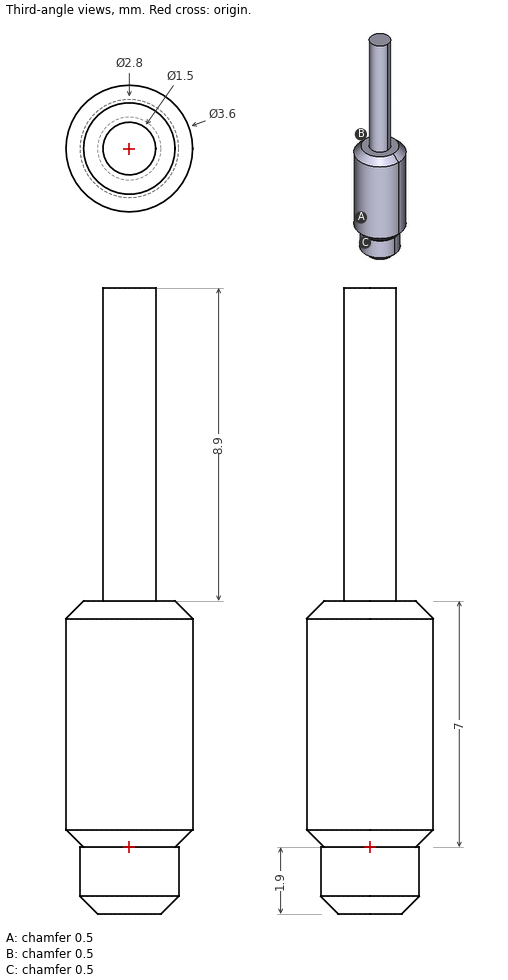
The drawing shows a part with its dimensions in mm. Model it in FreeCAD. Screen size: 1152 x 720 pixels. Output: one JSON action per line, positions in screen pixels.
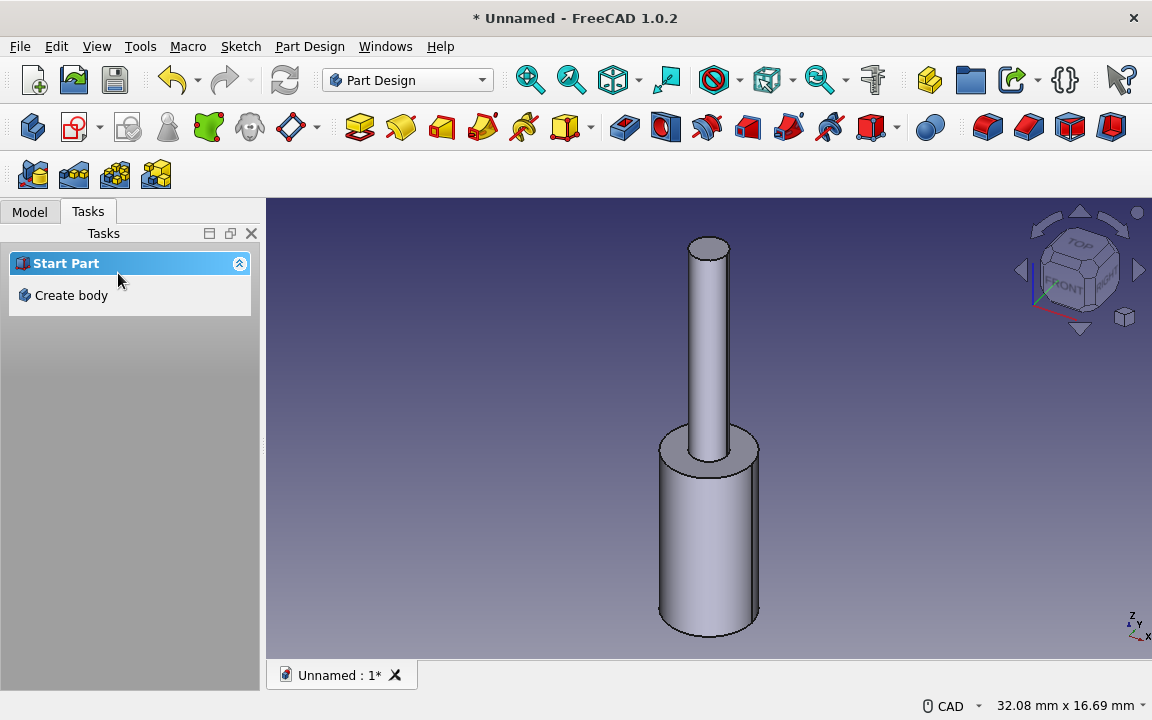
{"action": "key", "text": "0"}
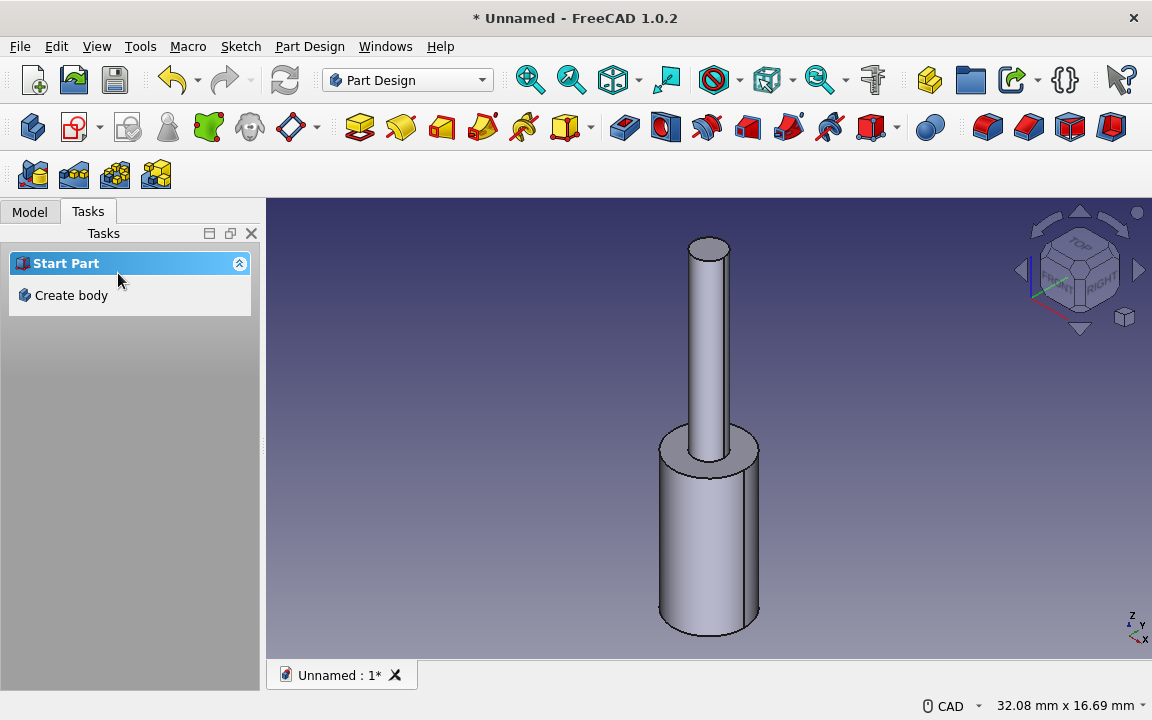
{"action": "key", "text": "2"}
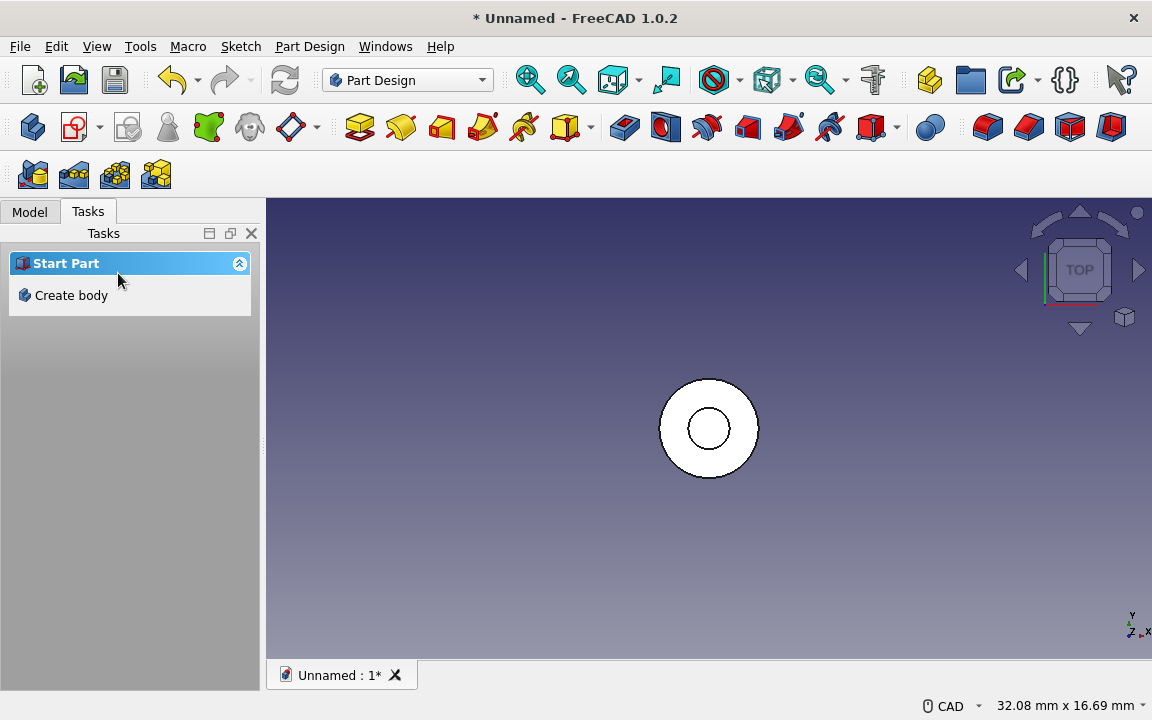
{"action": "key", "text": "v f"}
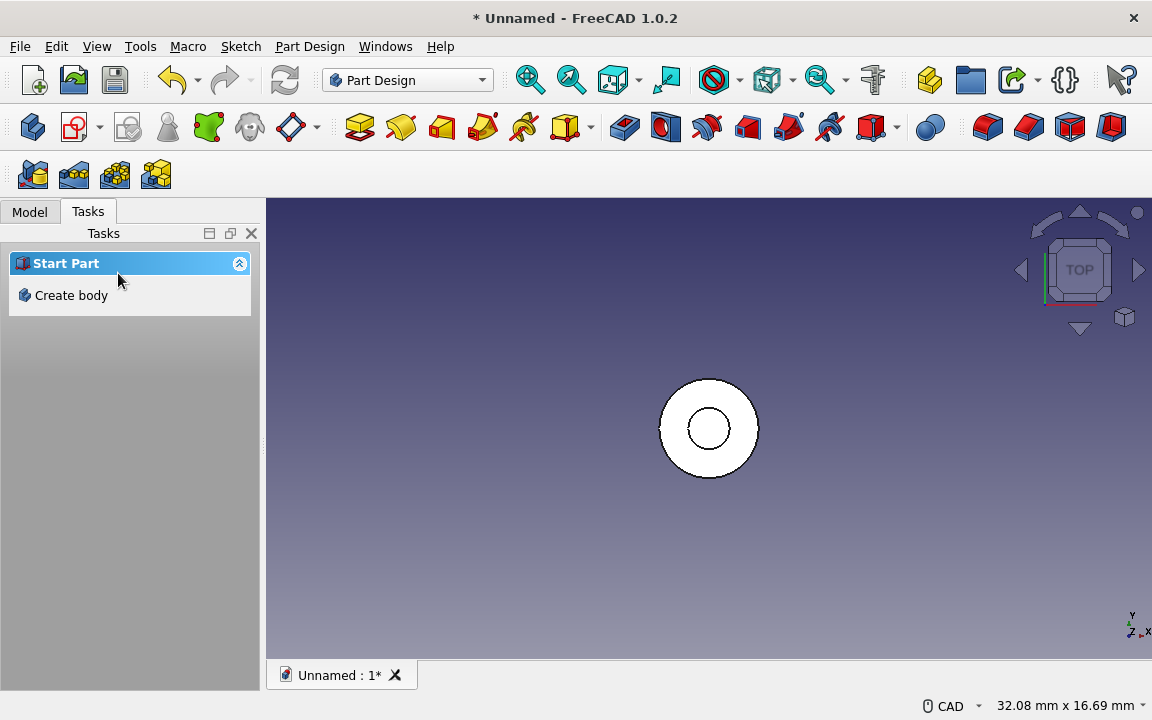
{"action": "key", "text": "1"}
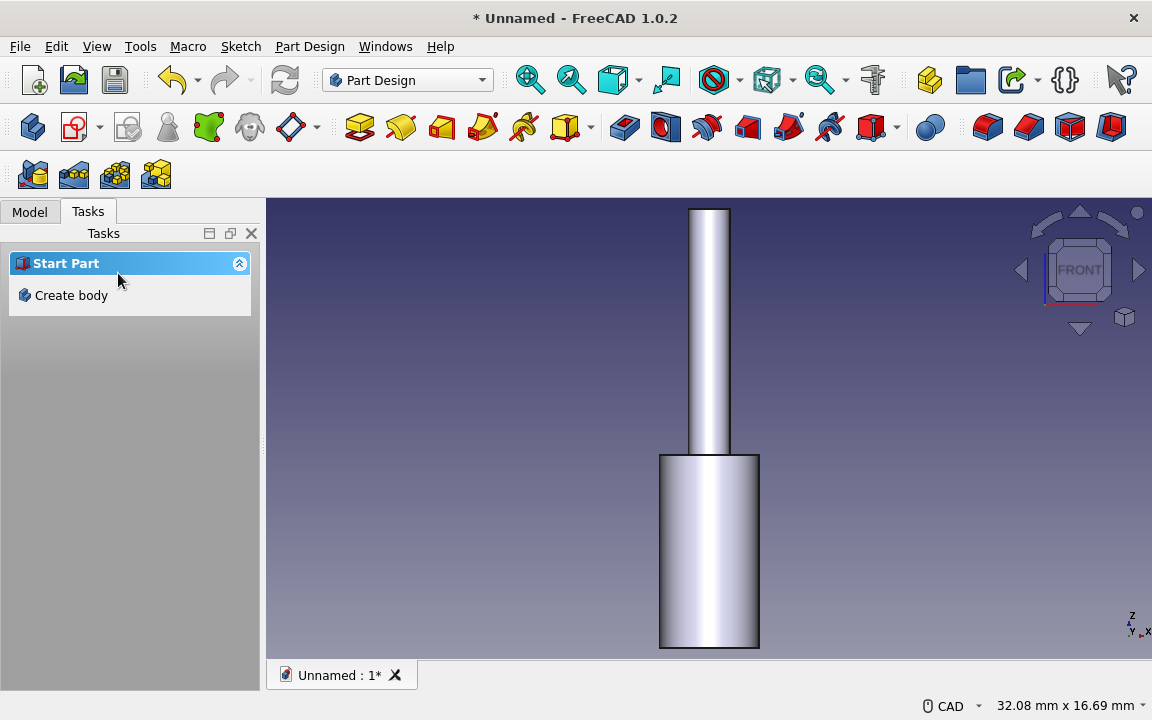
{"action": "key", "text": "3"}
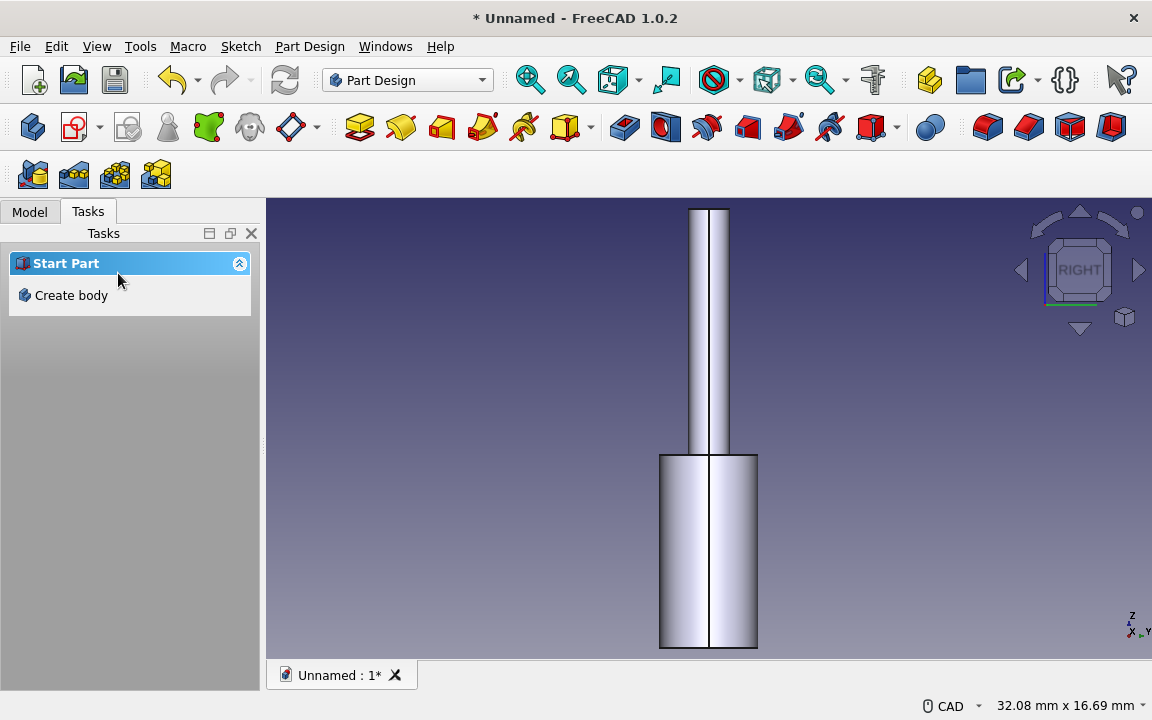
{"action": "key", "text": "5"}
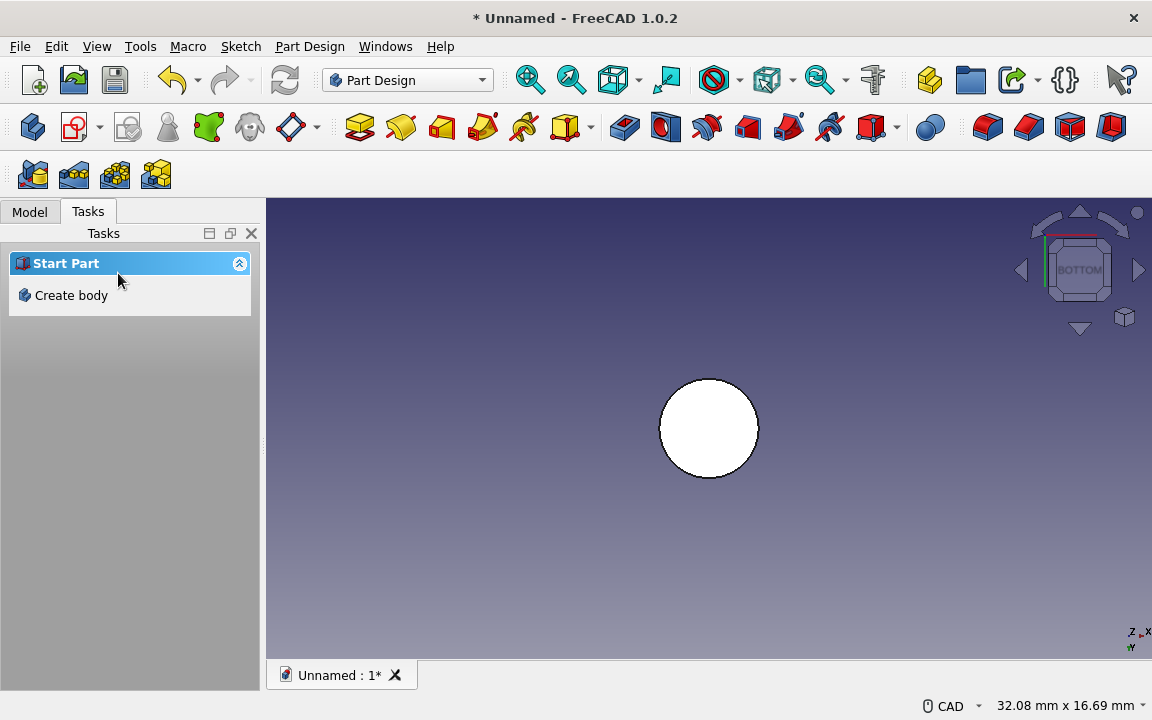
{"action": "left_click", "coordinate": [531, 80]}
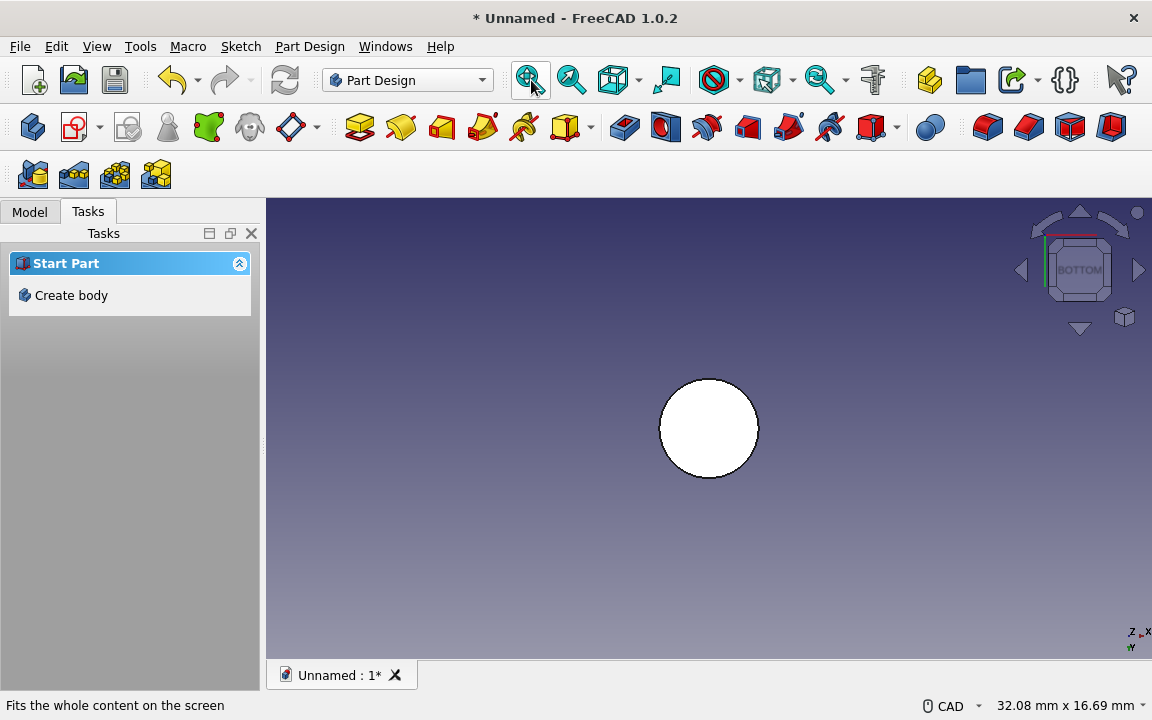
{"action": "left_click", "coordinate": [659, 427]}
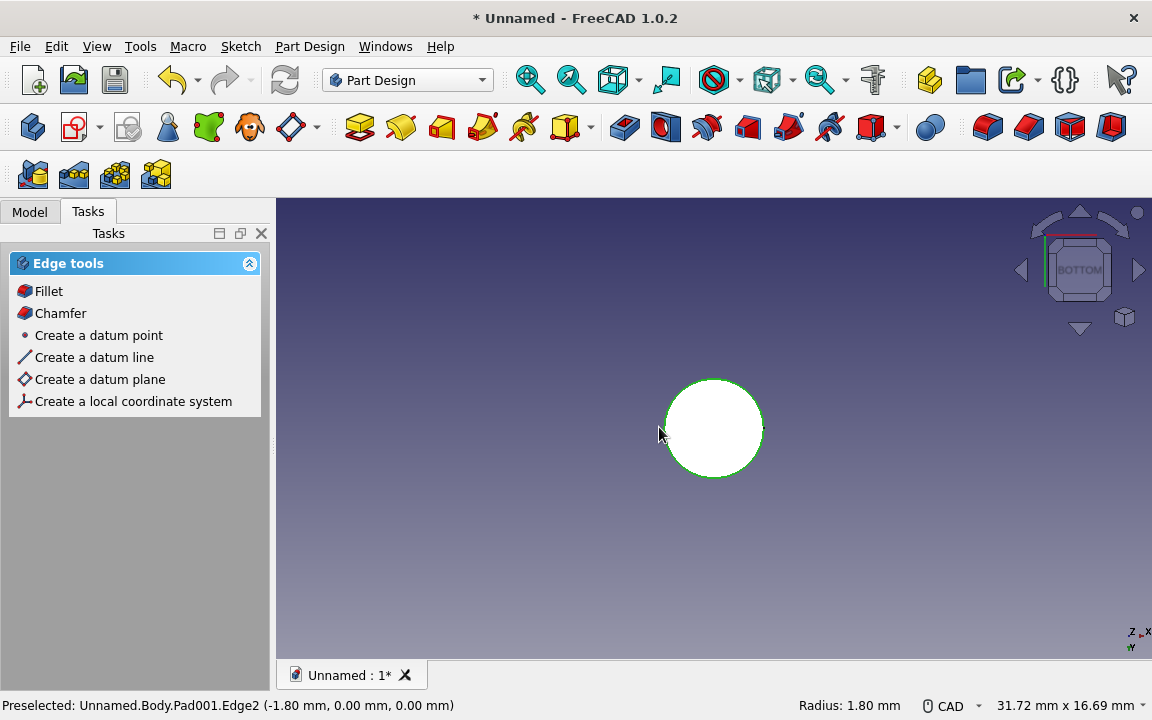
{"action": "left_click", "coordinate": [1029, 128]}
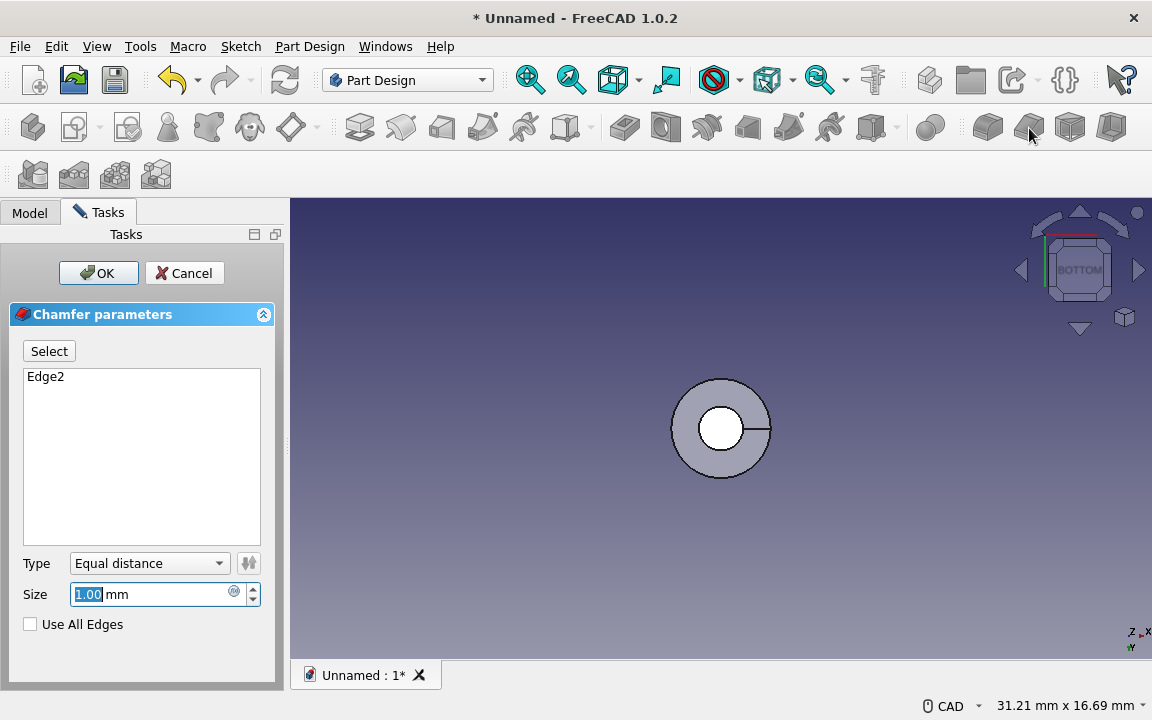
{"action": "type", "text": "0.5"}
{"action": "key", "text": "Tab"}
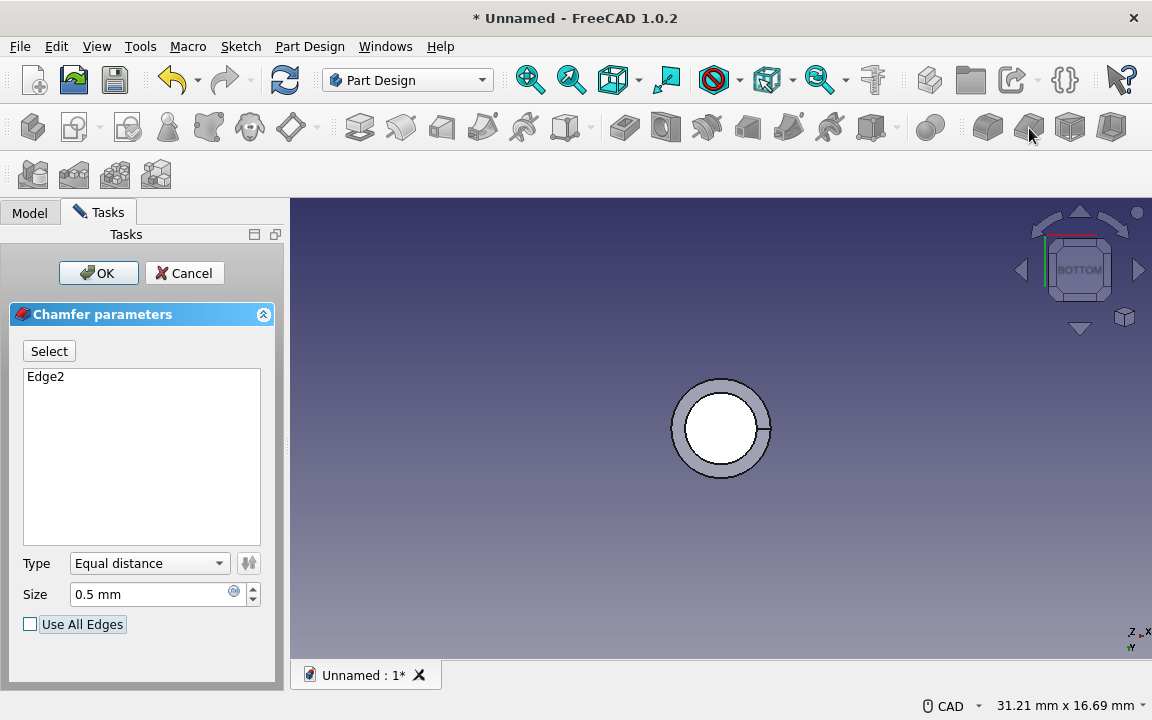
{"action": "left_click", "coordinate": [99, 273]}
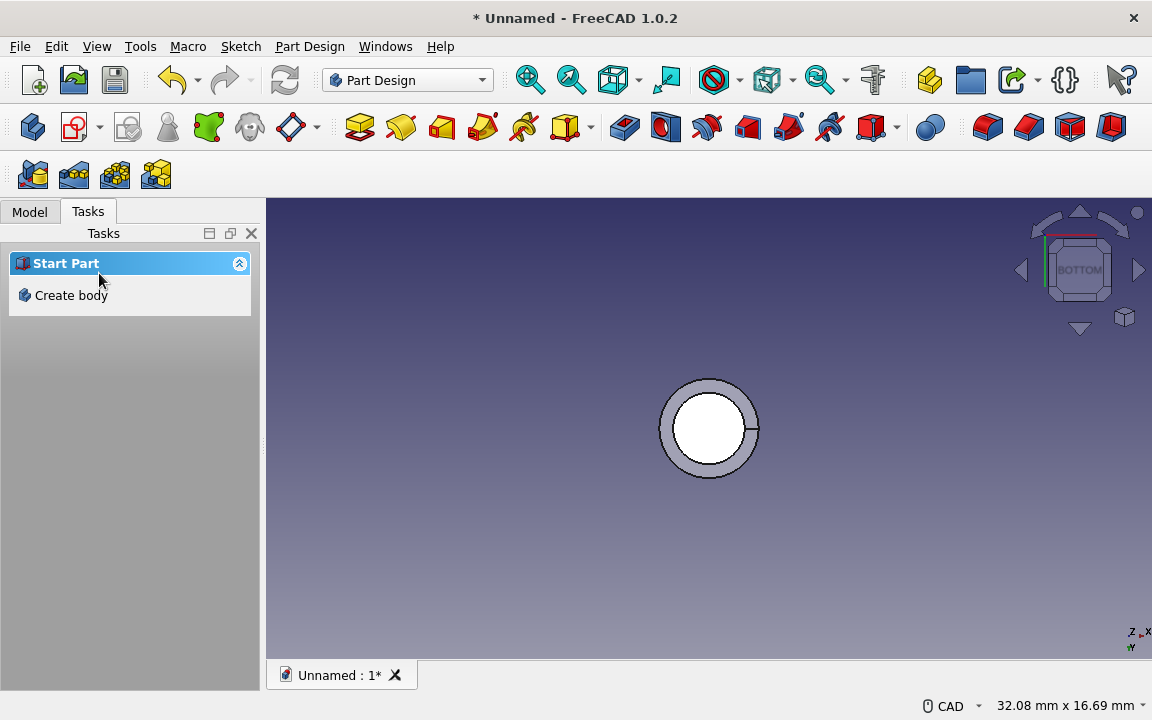
{"action": "key", "text": "v f"}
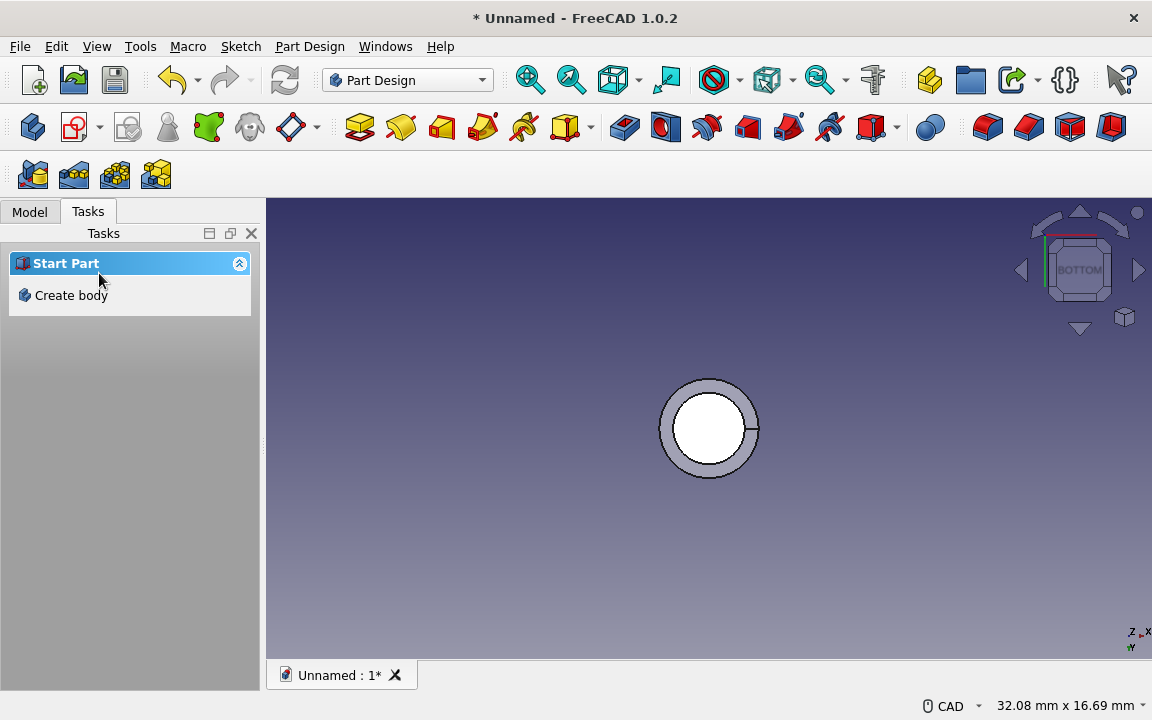
{"action": "key", "text": "0"}